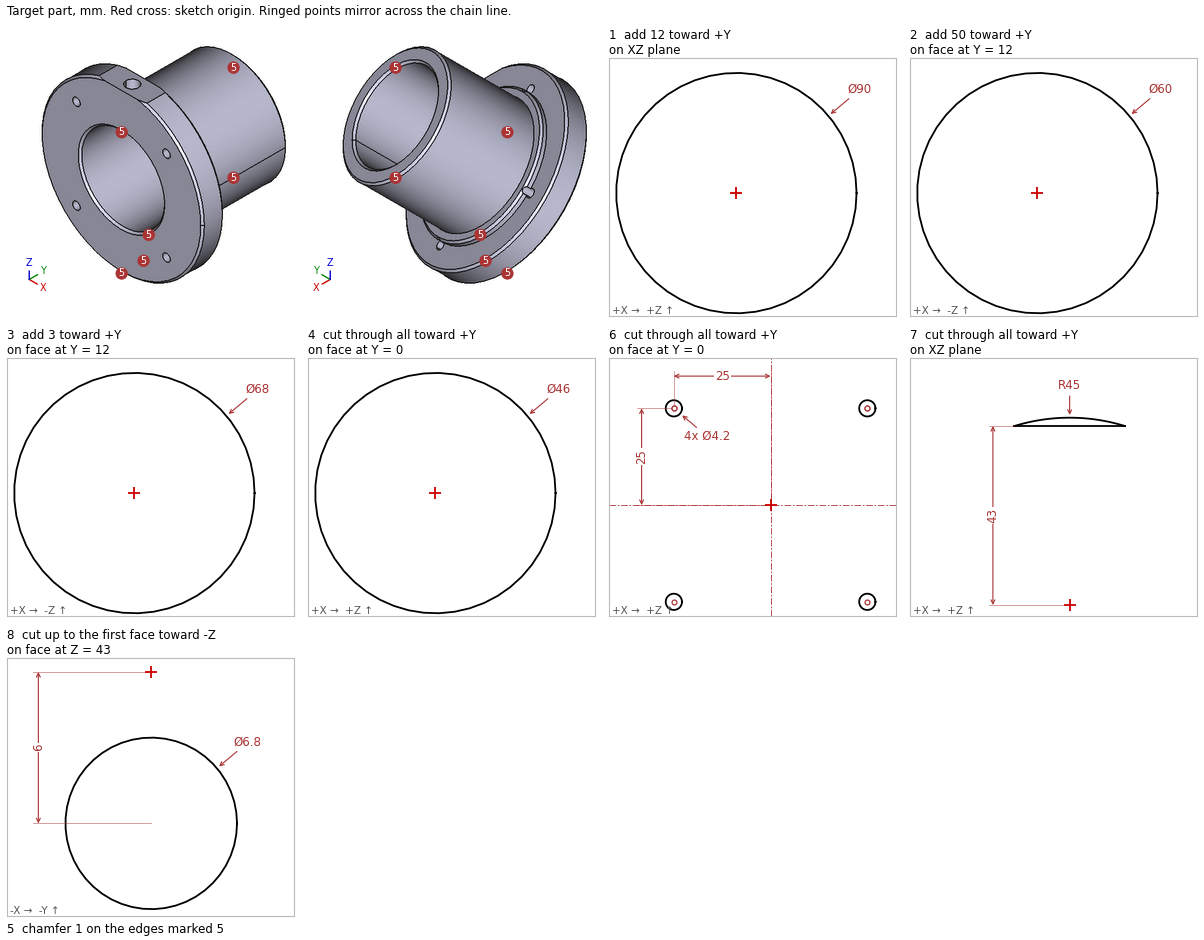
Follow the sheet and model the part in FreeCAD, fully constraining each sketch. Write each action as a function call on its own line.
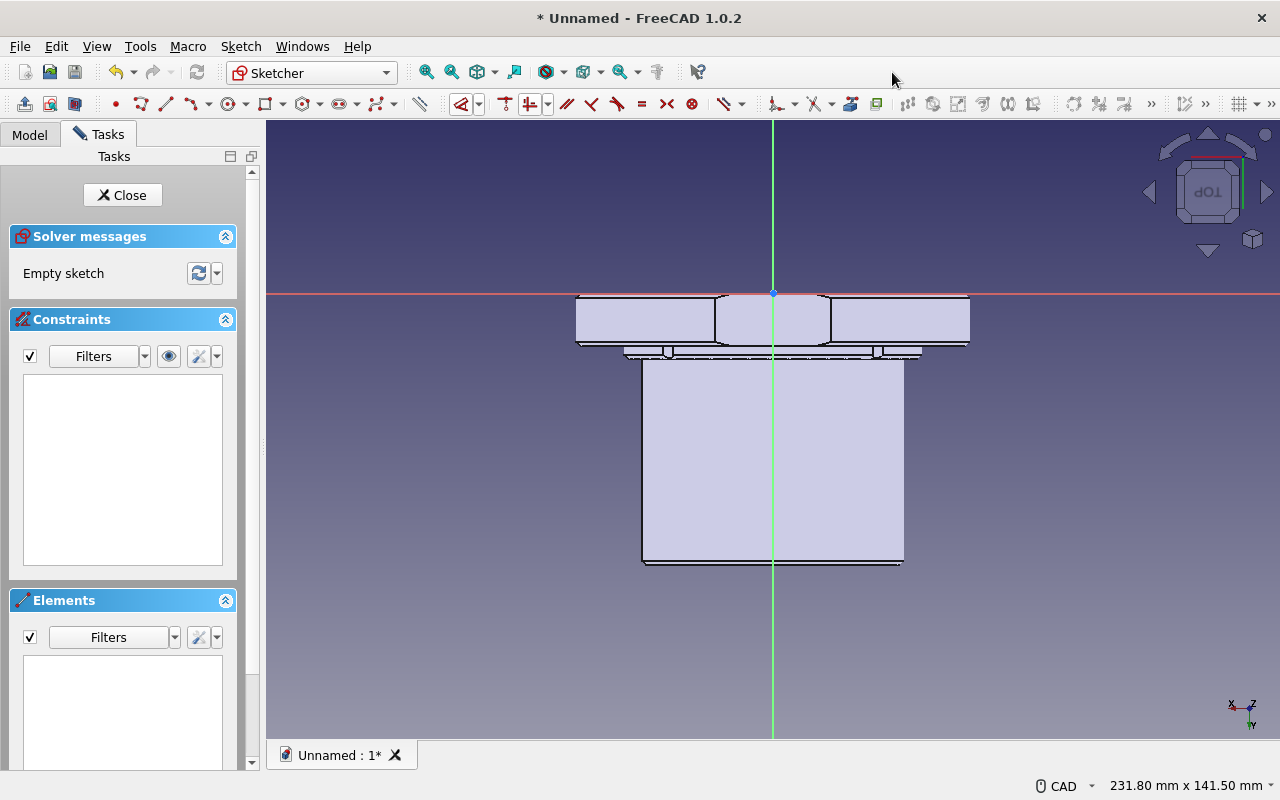
scroll(782, 300, up, 11)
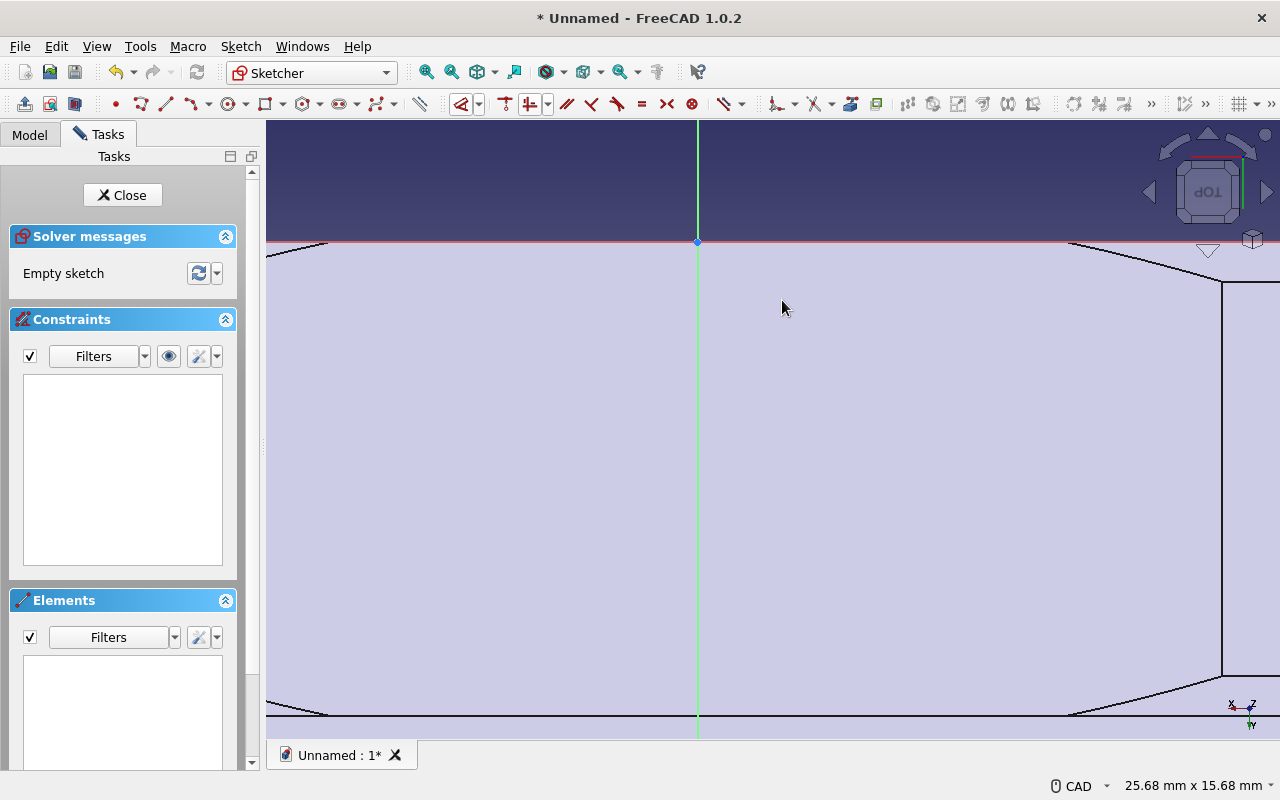
click(228, 104)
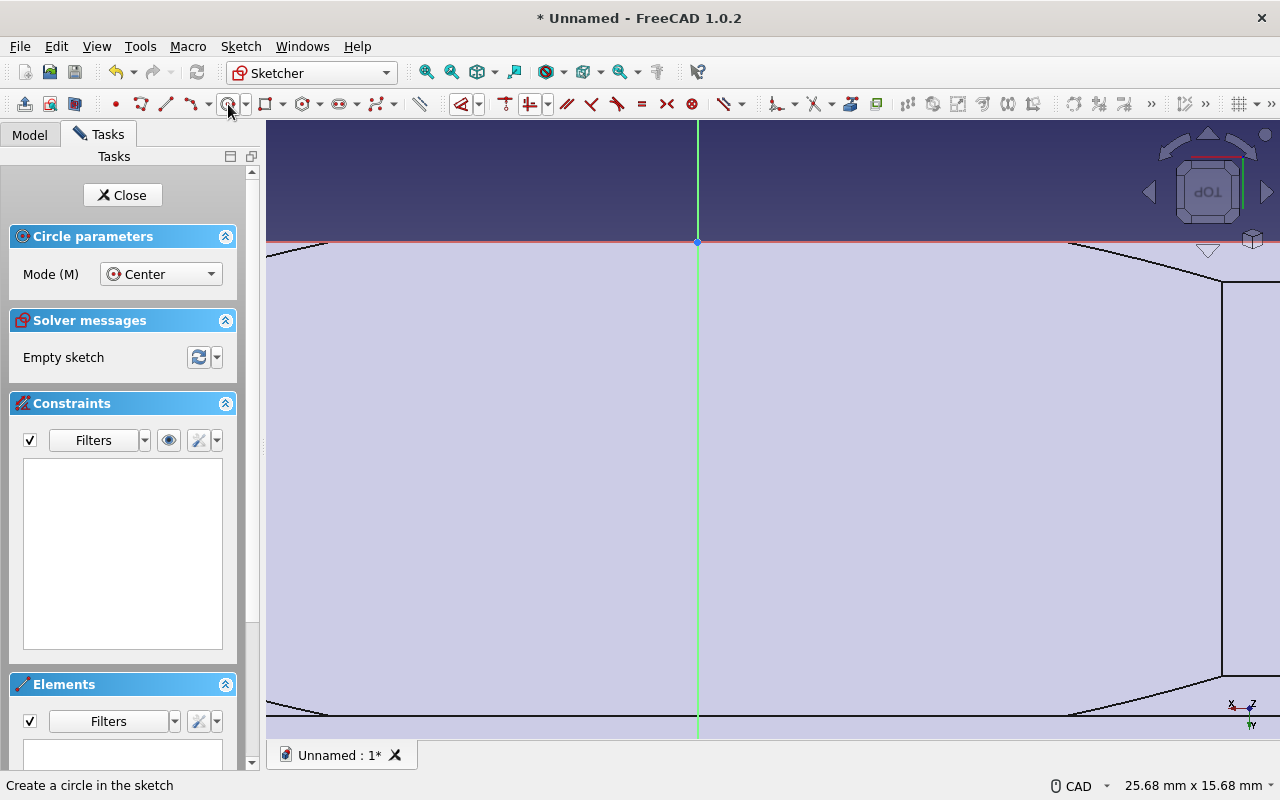
click(698, 479)
move(793, 384)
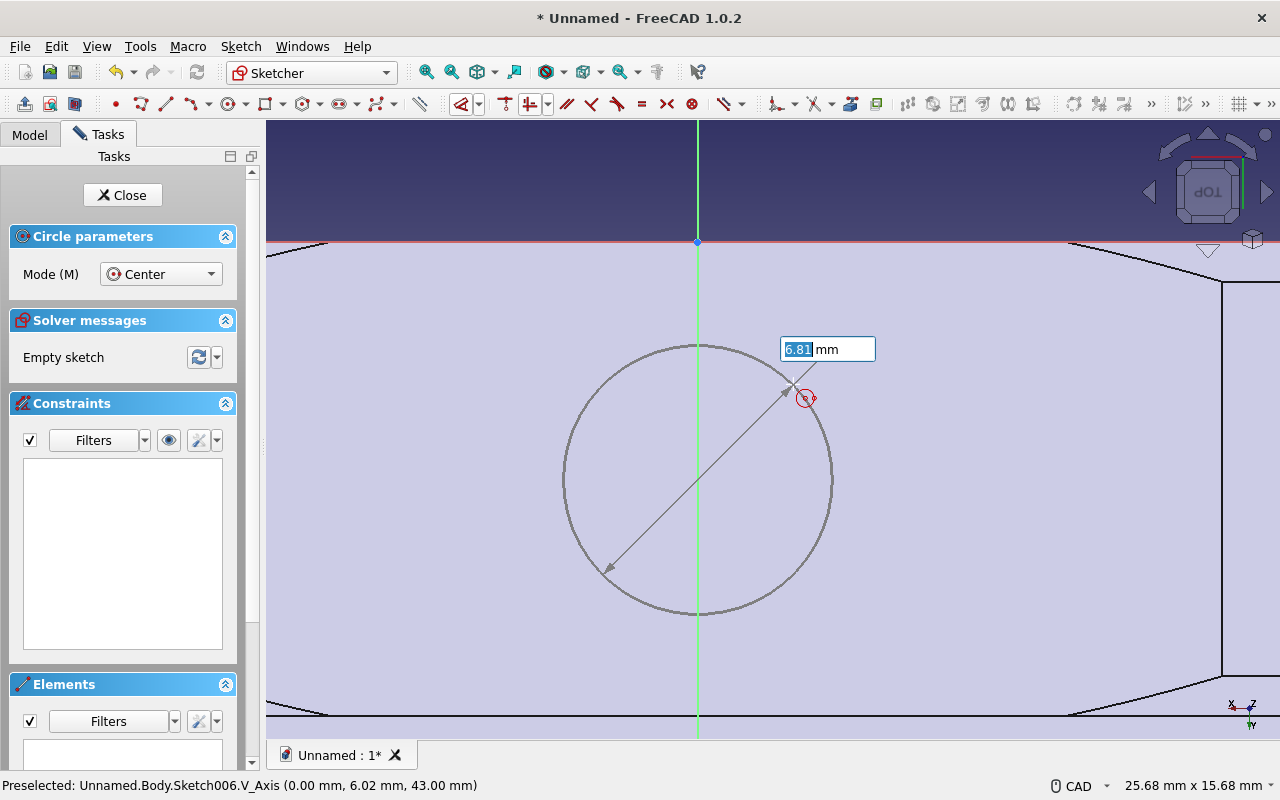
text(6.8)
key(Return)
key(Escape)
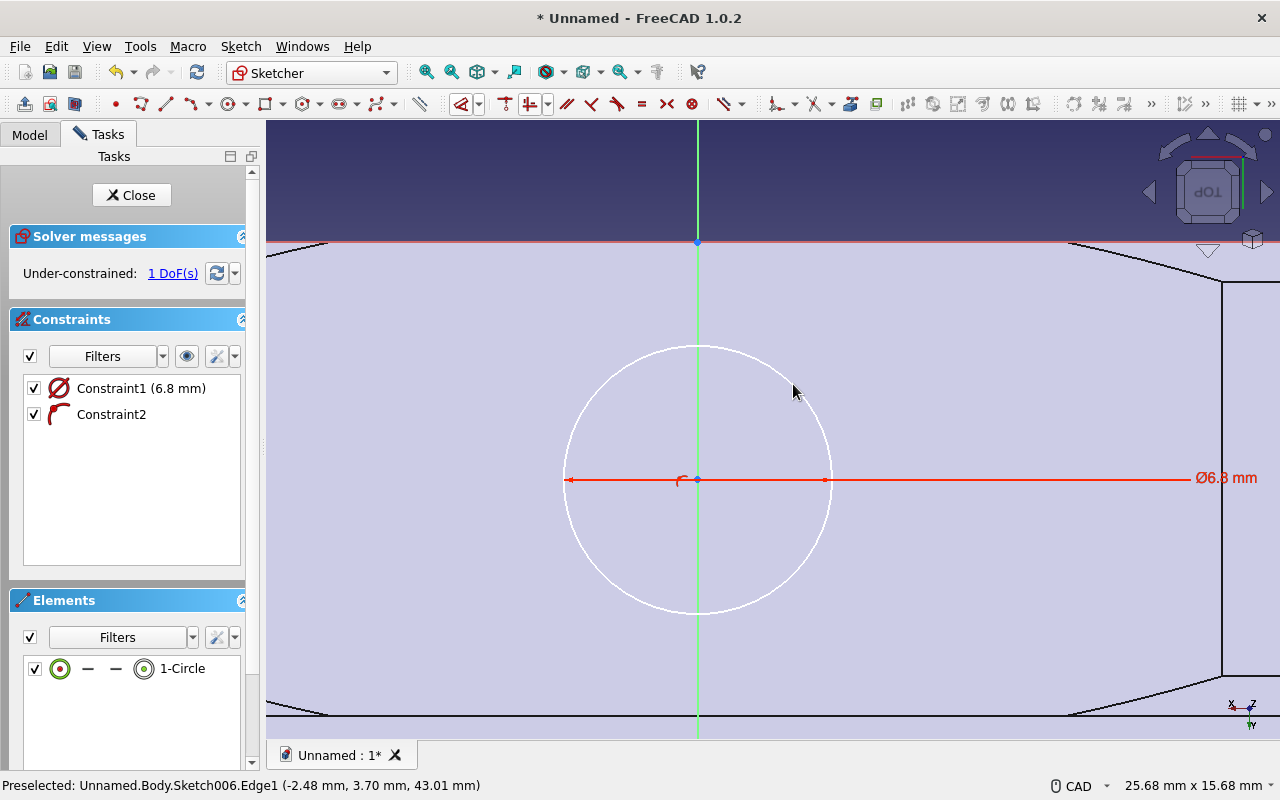
click(698, 480)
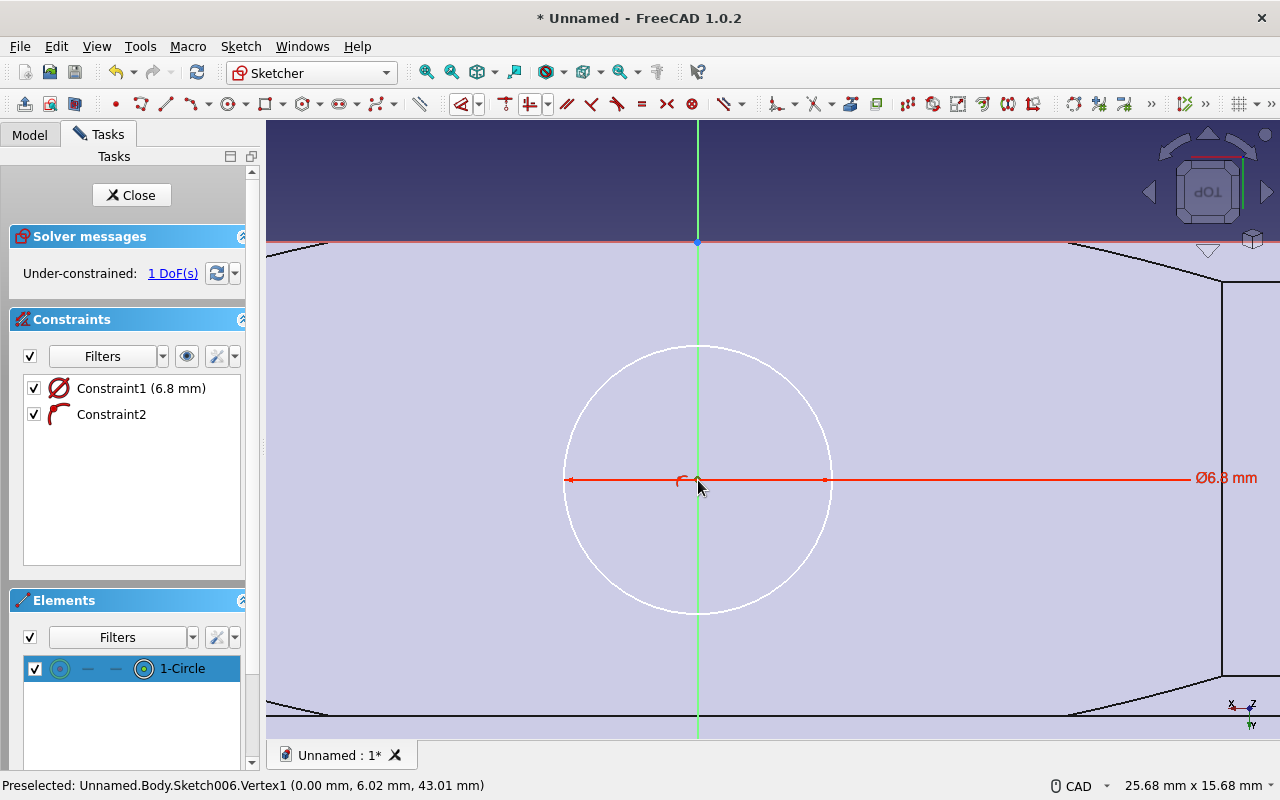
key(i)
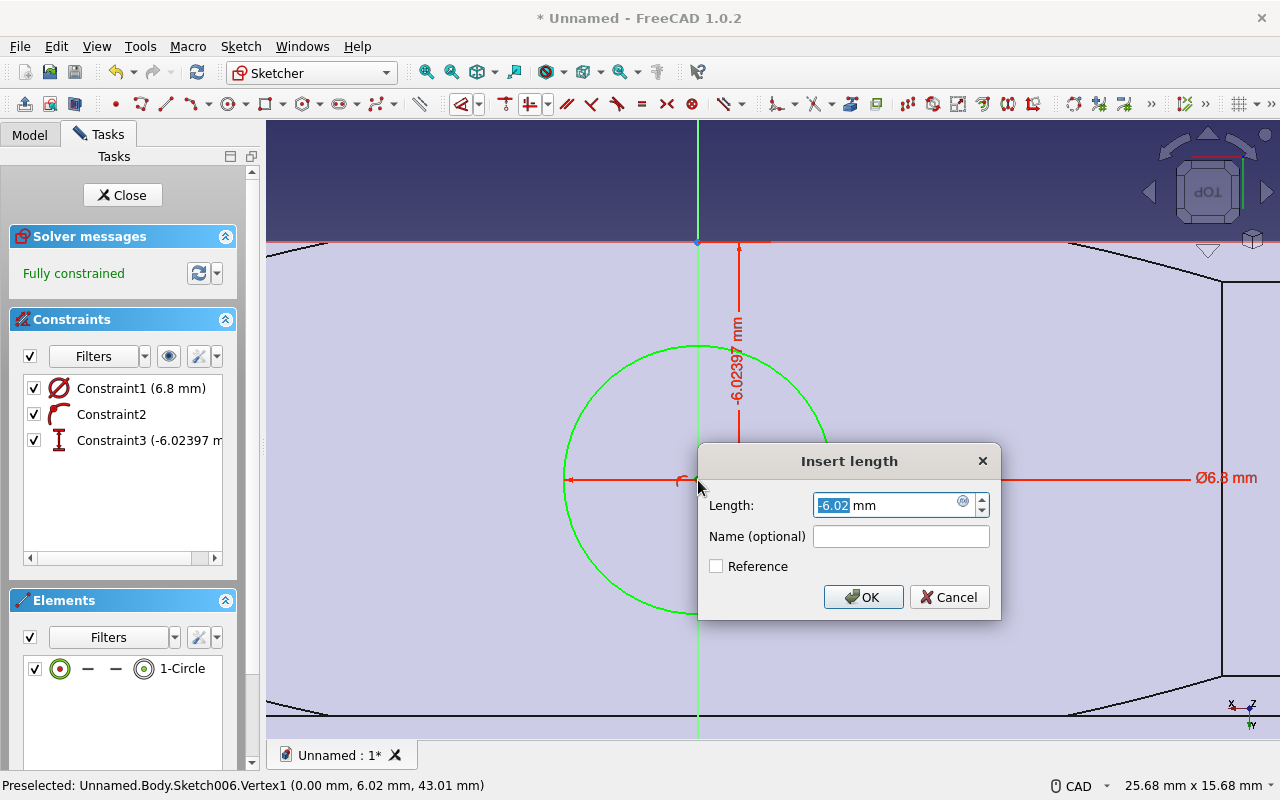
text(-6)
key(Return)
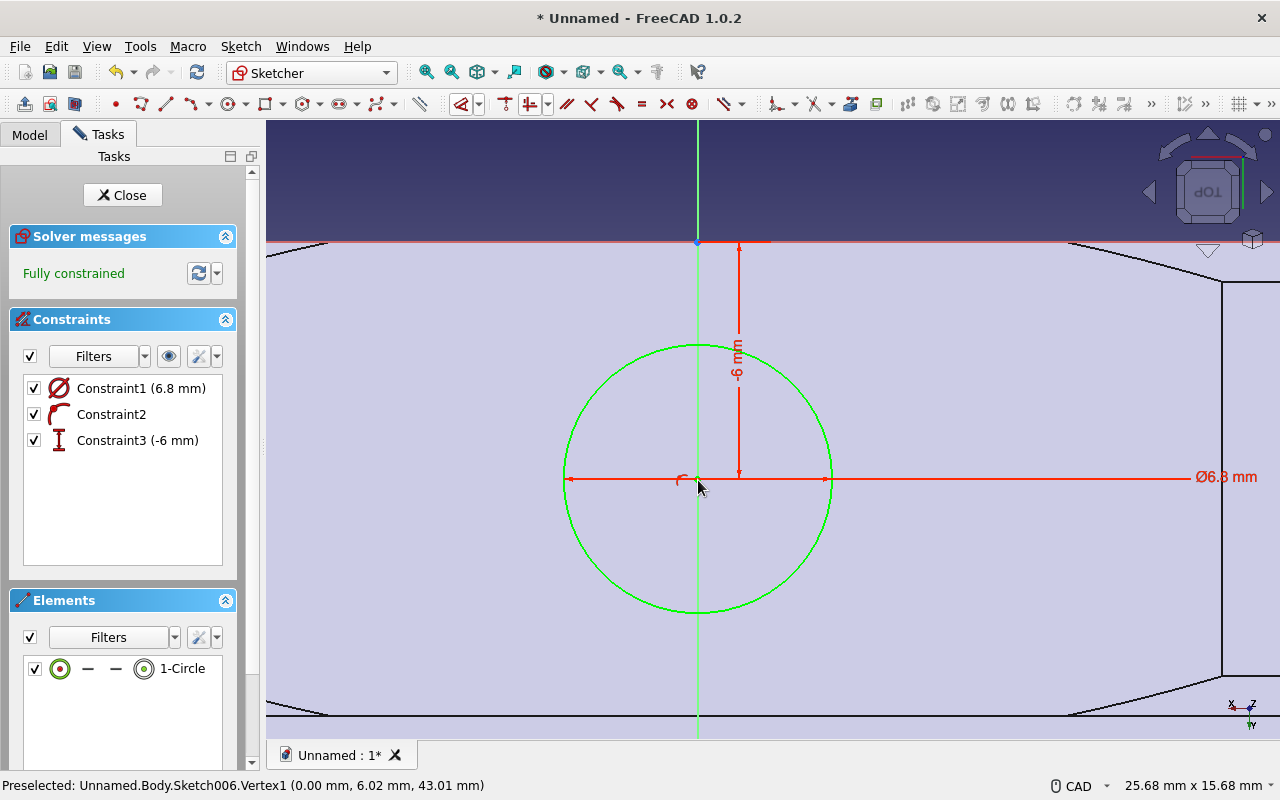
click(123, 195)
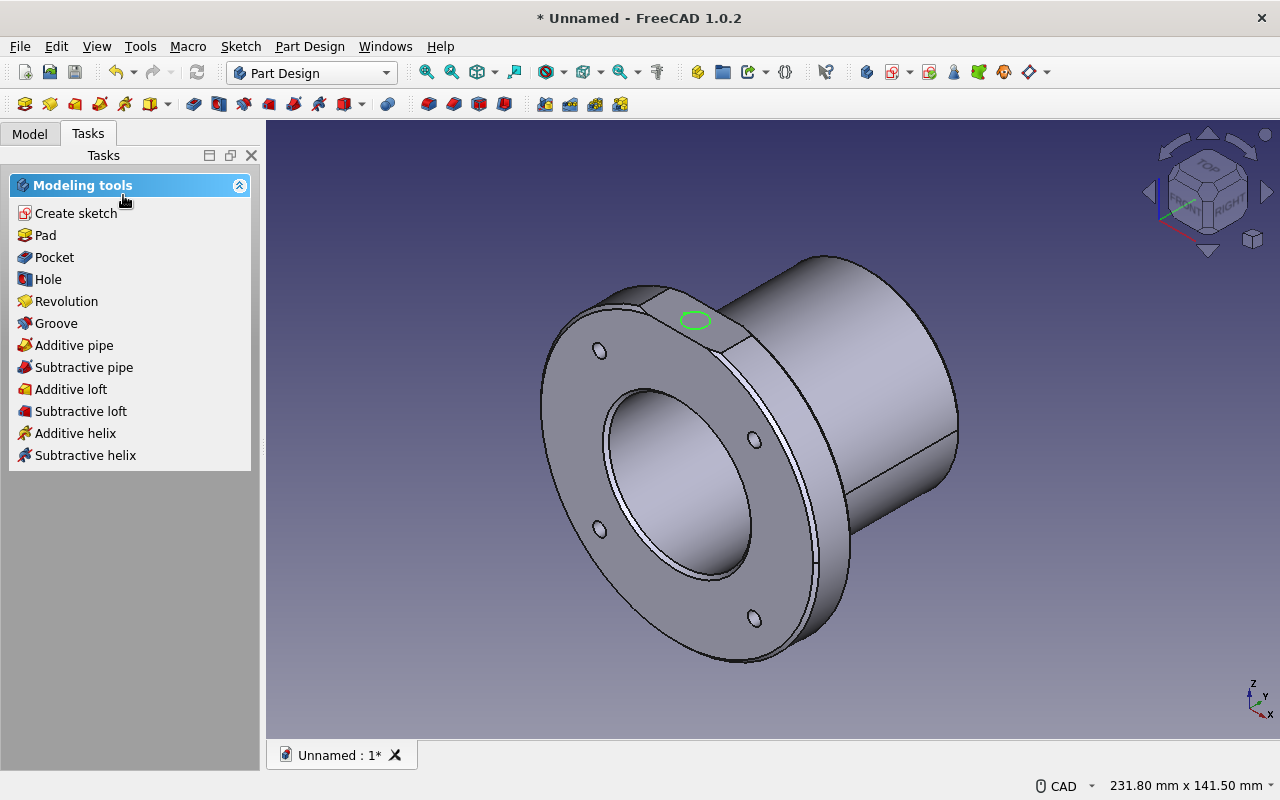
click(194, 104)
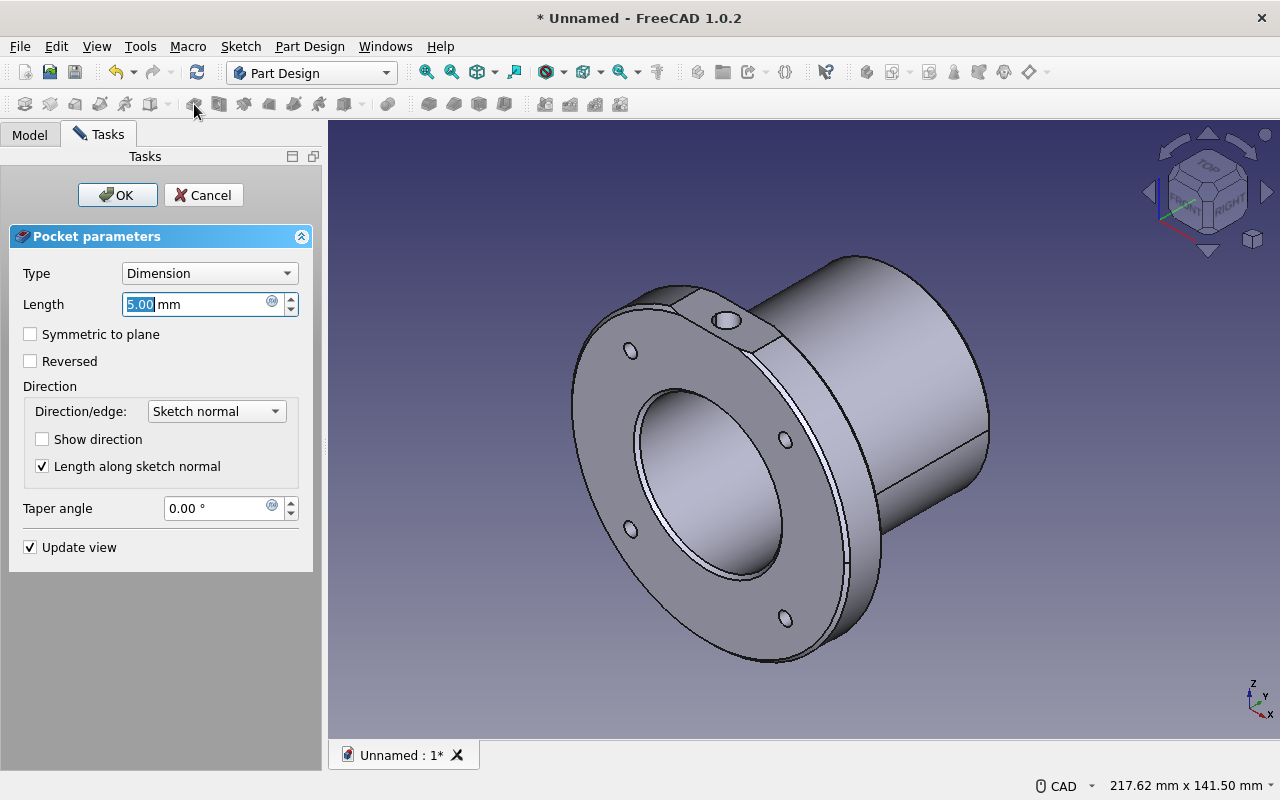
click(210, 274)